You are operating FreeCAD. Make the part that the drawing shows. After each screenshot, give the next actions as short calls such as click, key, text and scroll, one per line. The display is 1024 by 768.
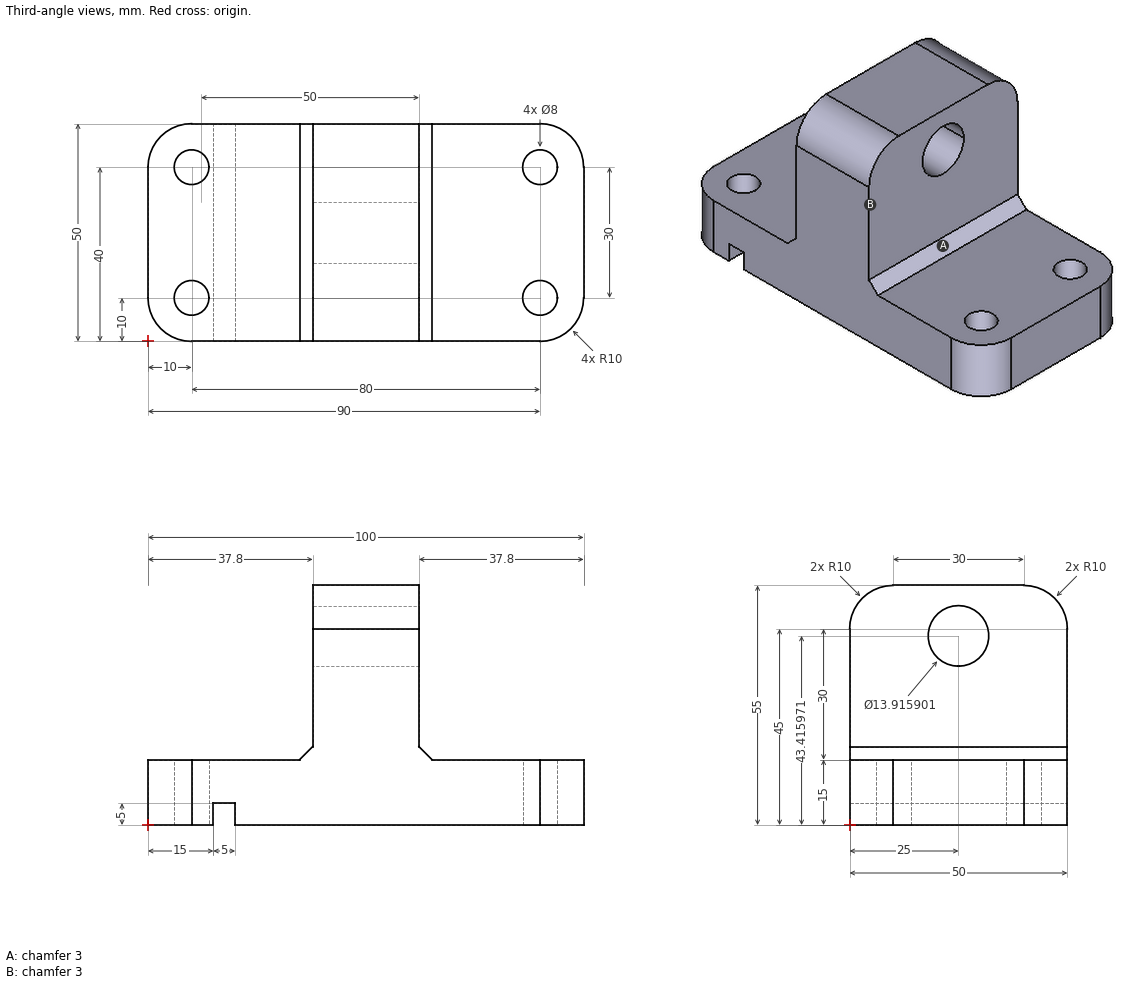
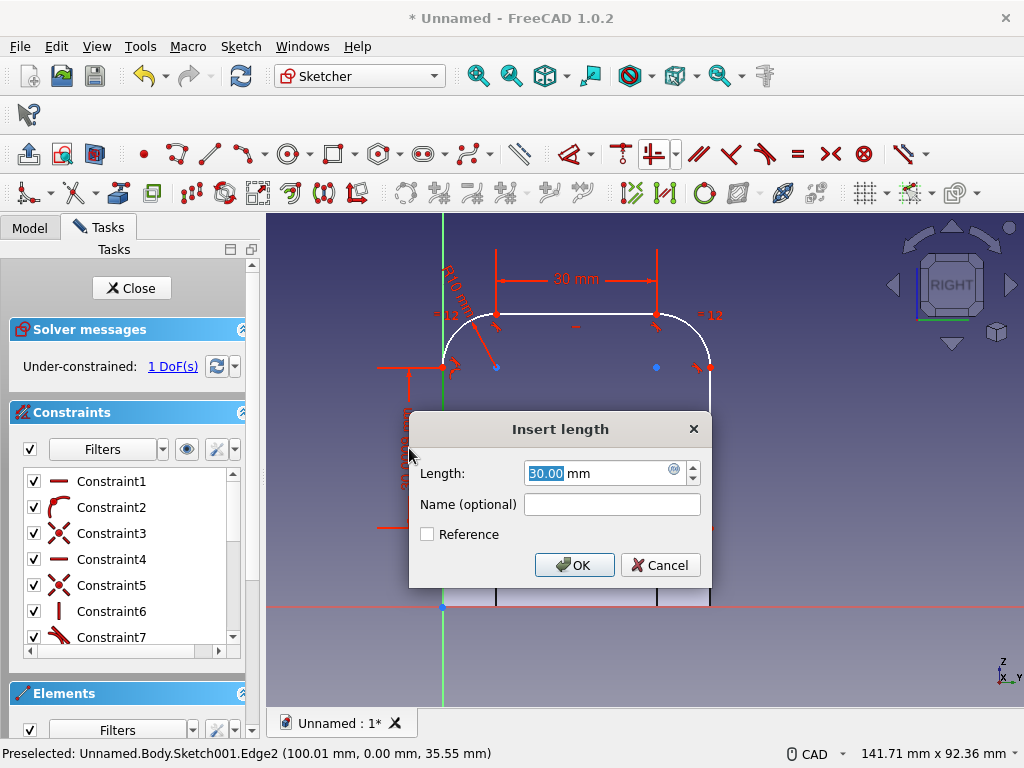
text(30)
key(Return)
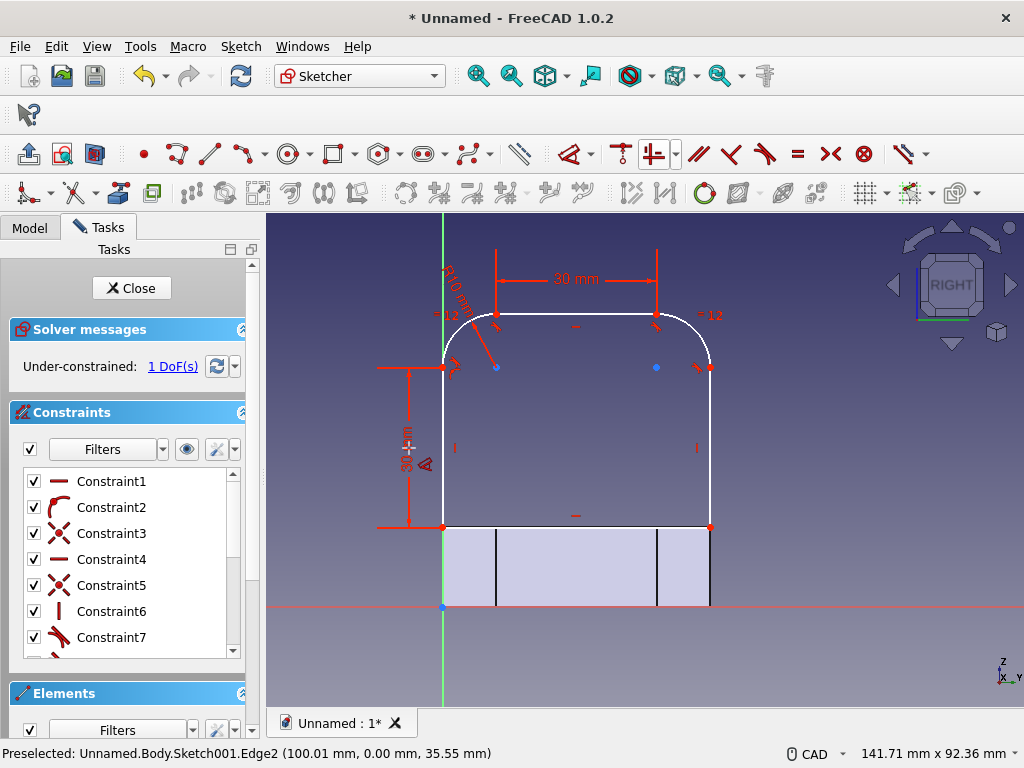
click(657, 314)
click(409, 393)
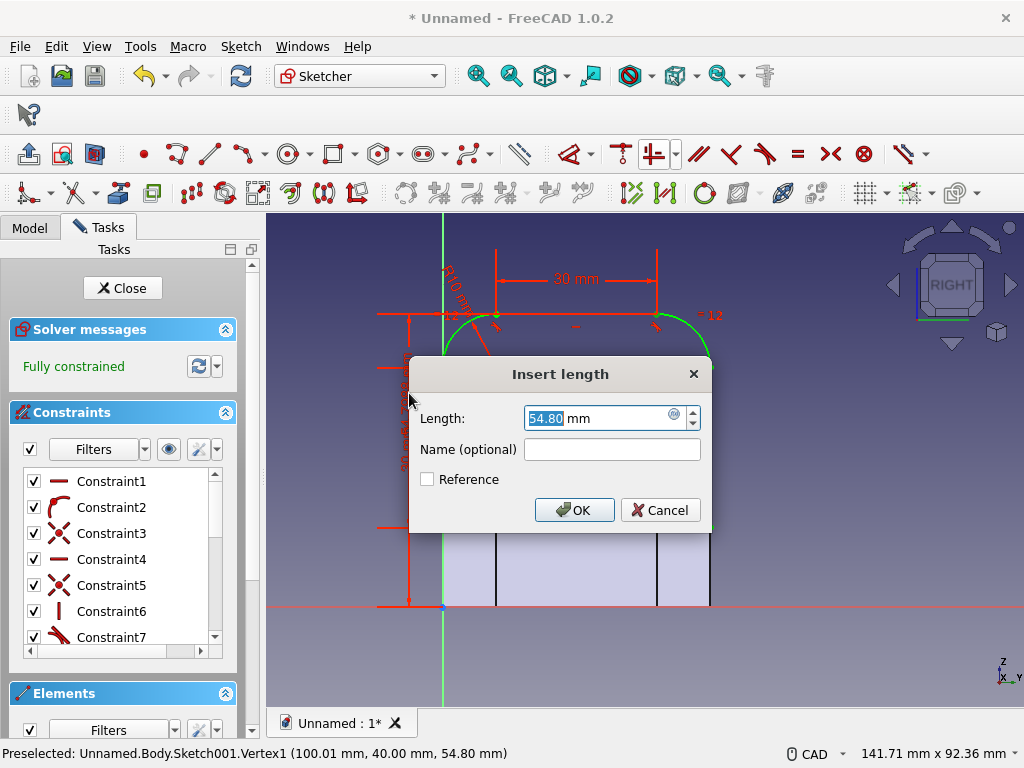
text(55)
key(Return)
key(Escape)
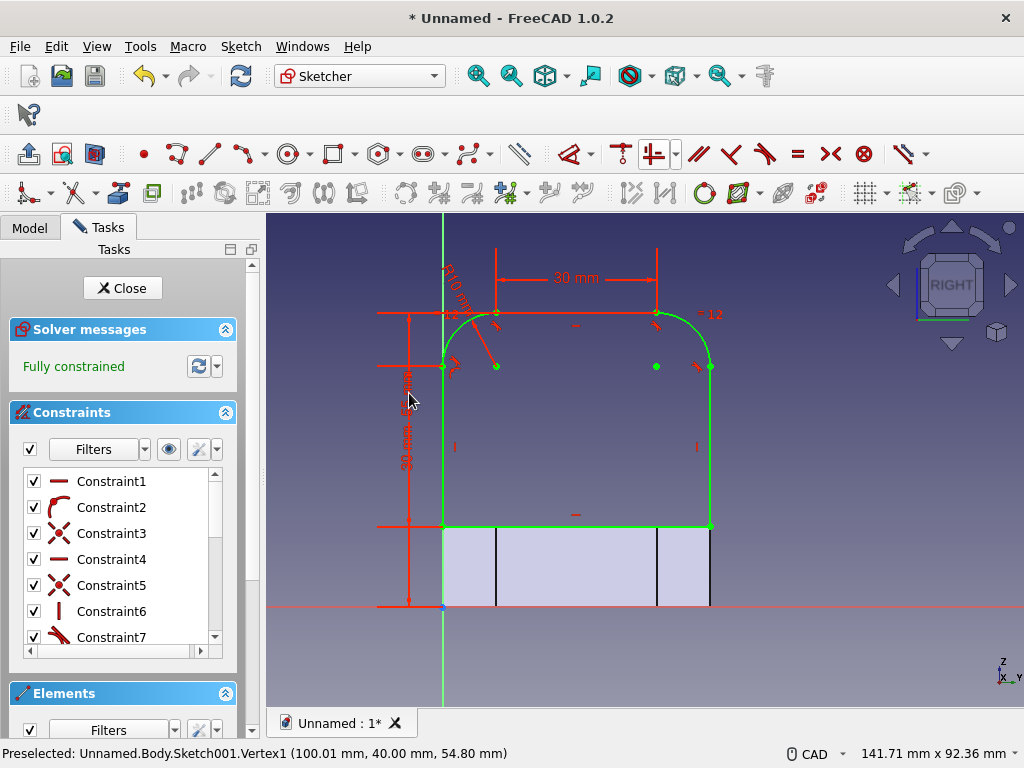
click(123, 288)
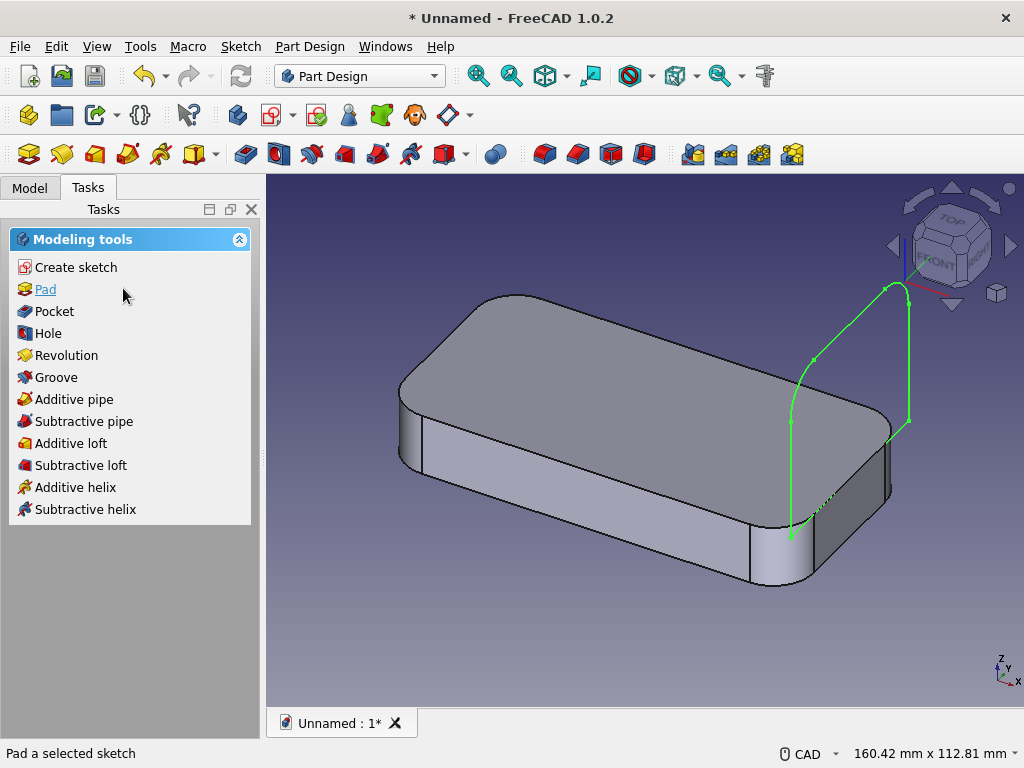
click(29, 154)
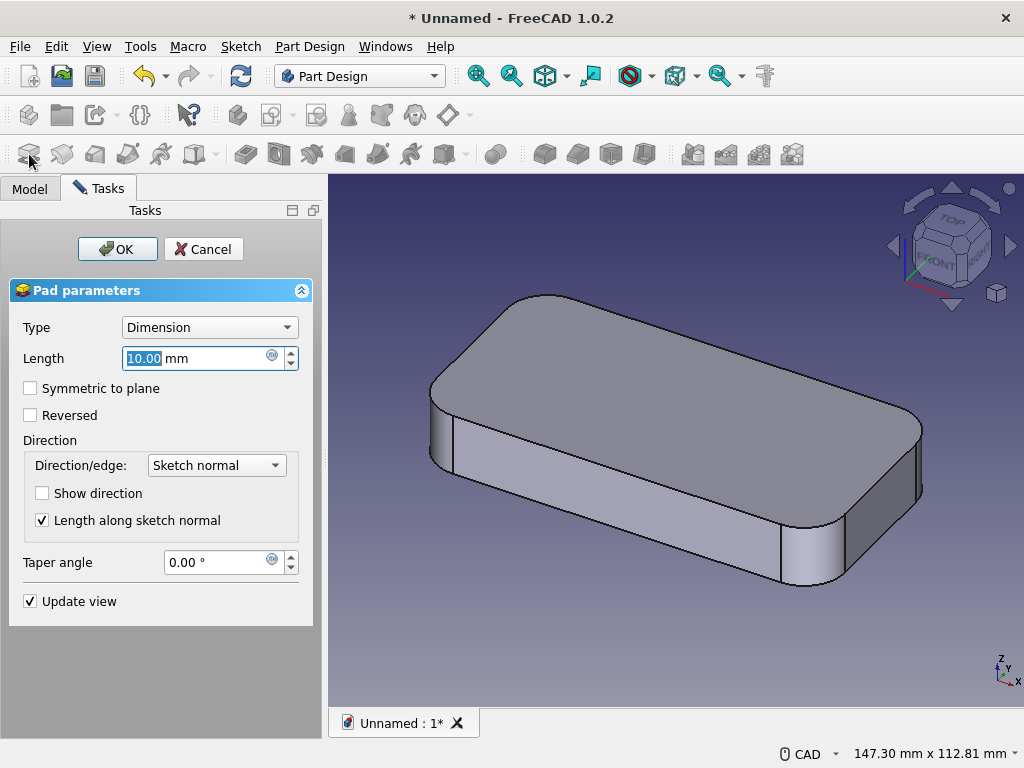
text(100)
key(Tab)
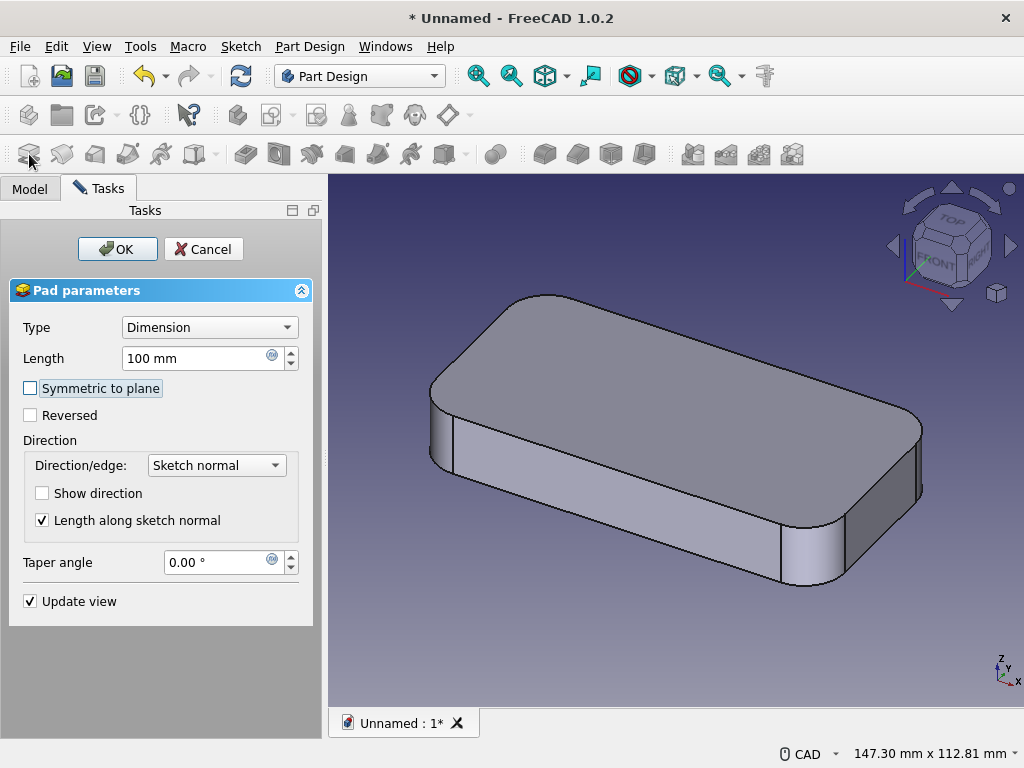
click(31, 415)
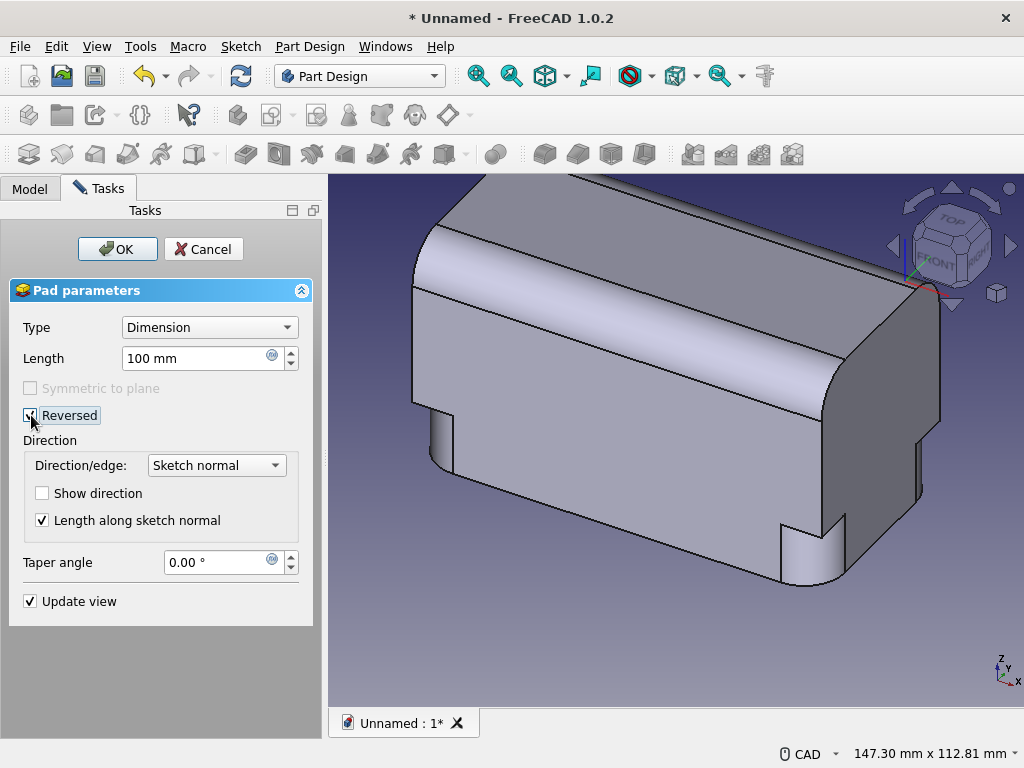
click(118, 249)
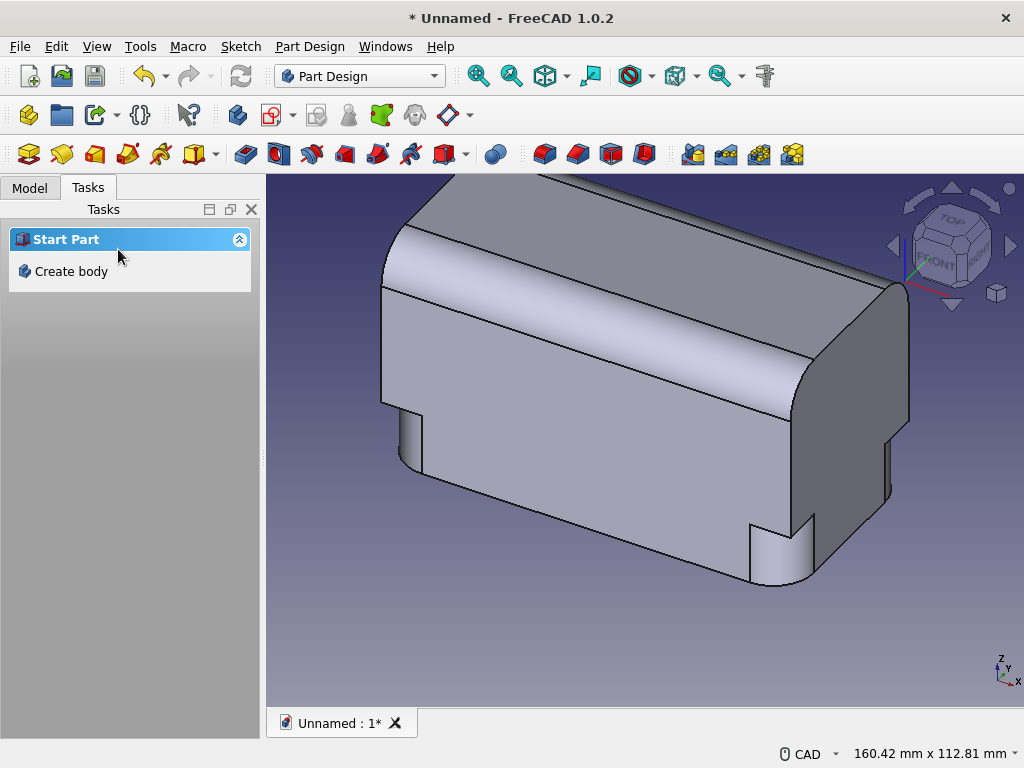
click(479, 76)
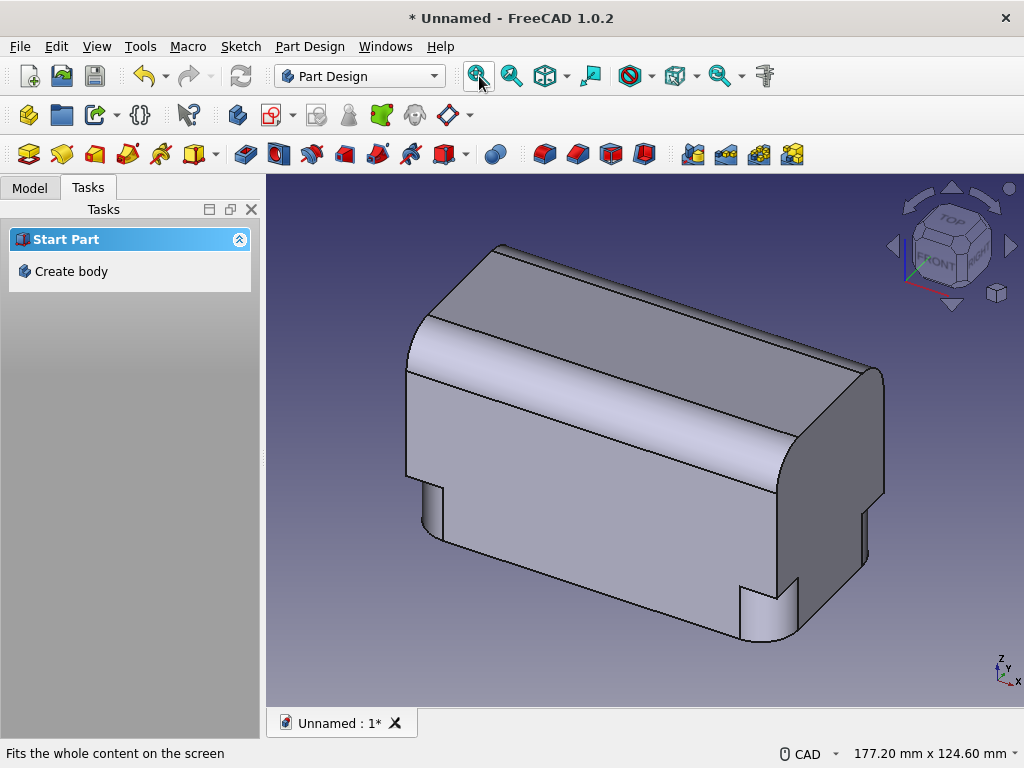
click(830, 473)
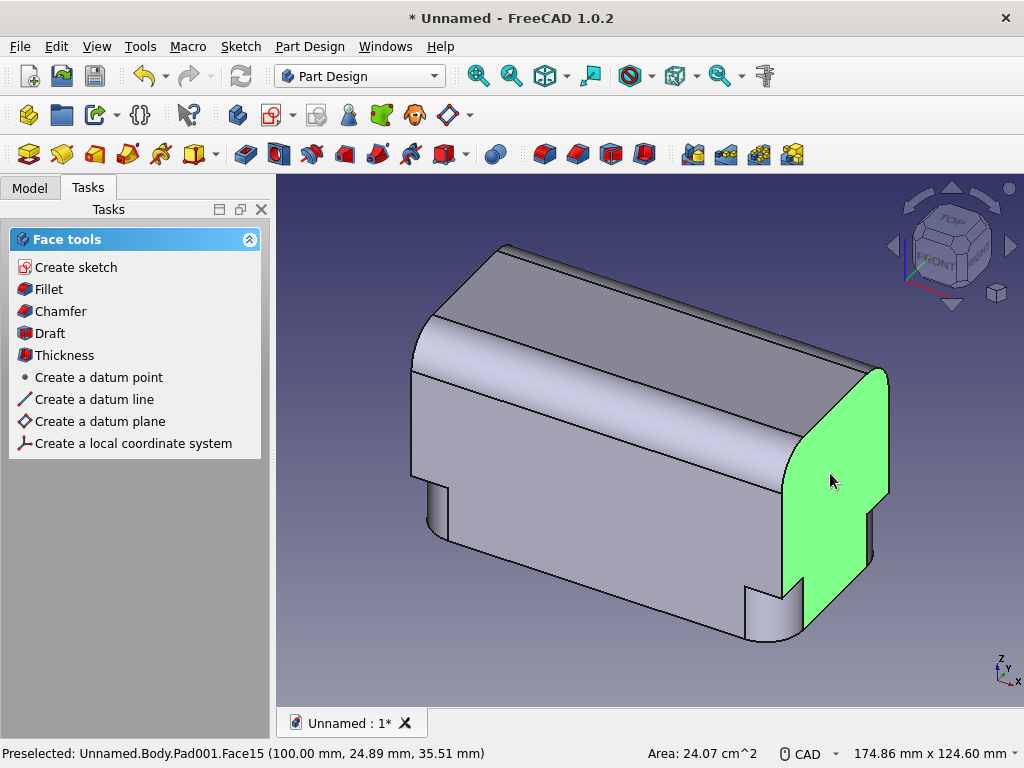
click(270, 116)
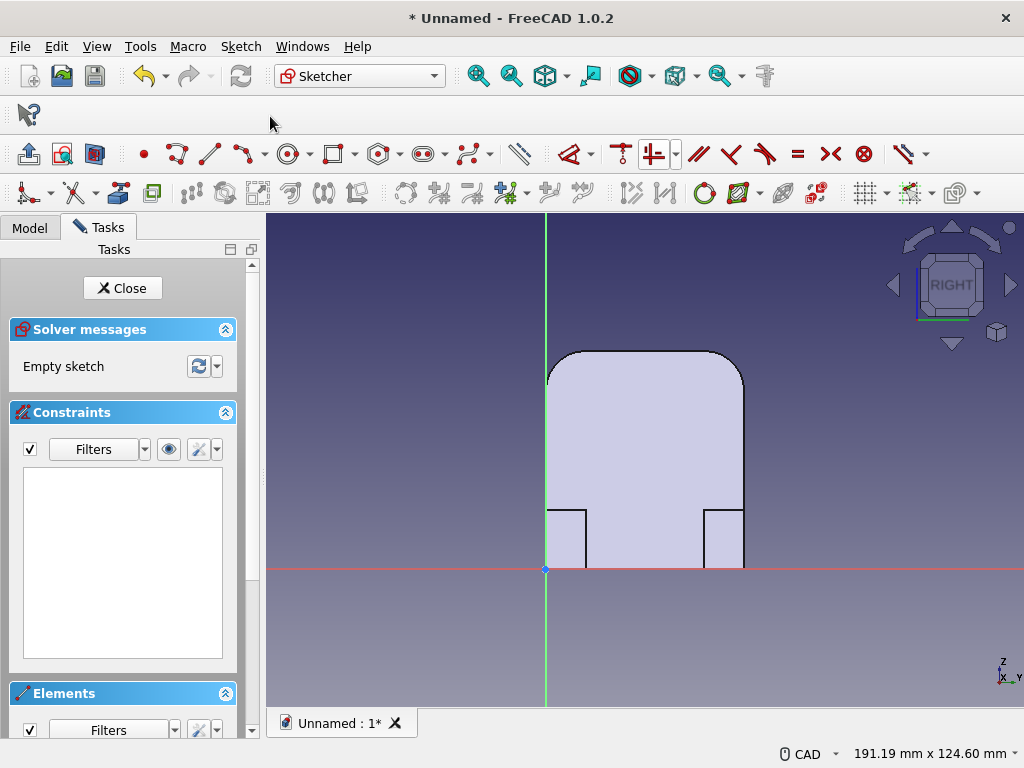
scroll(784, 460, up, 2)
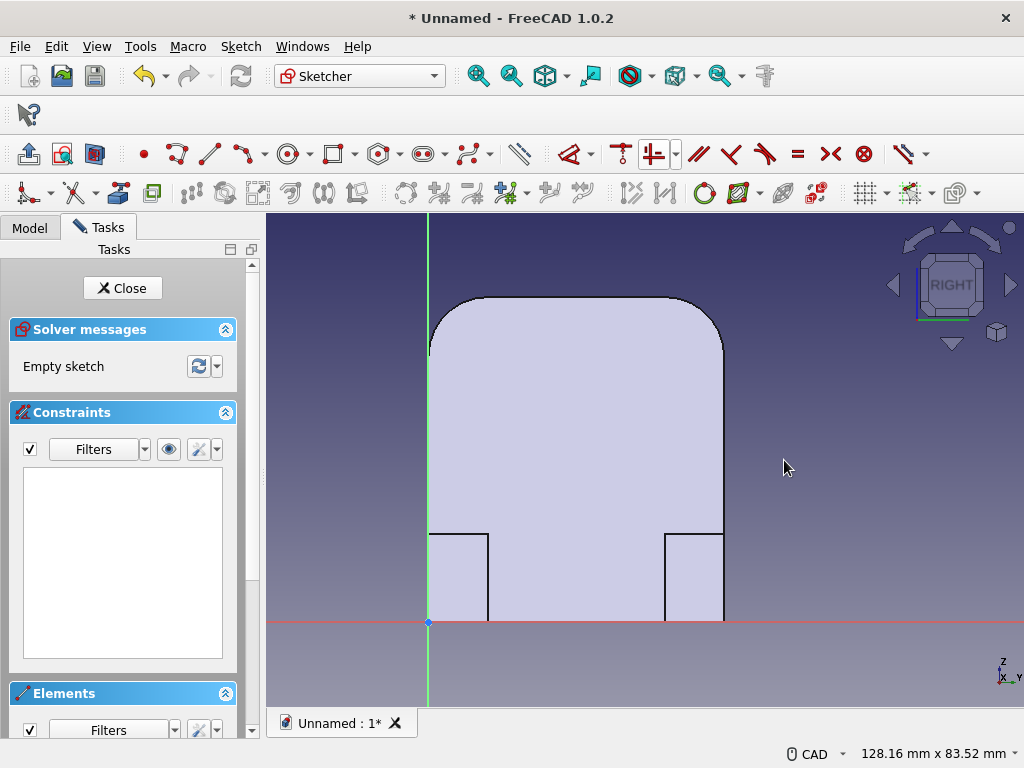
click(210, 154)